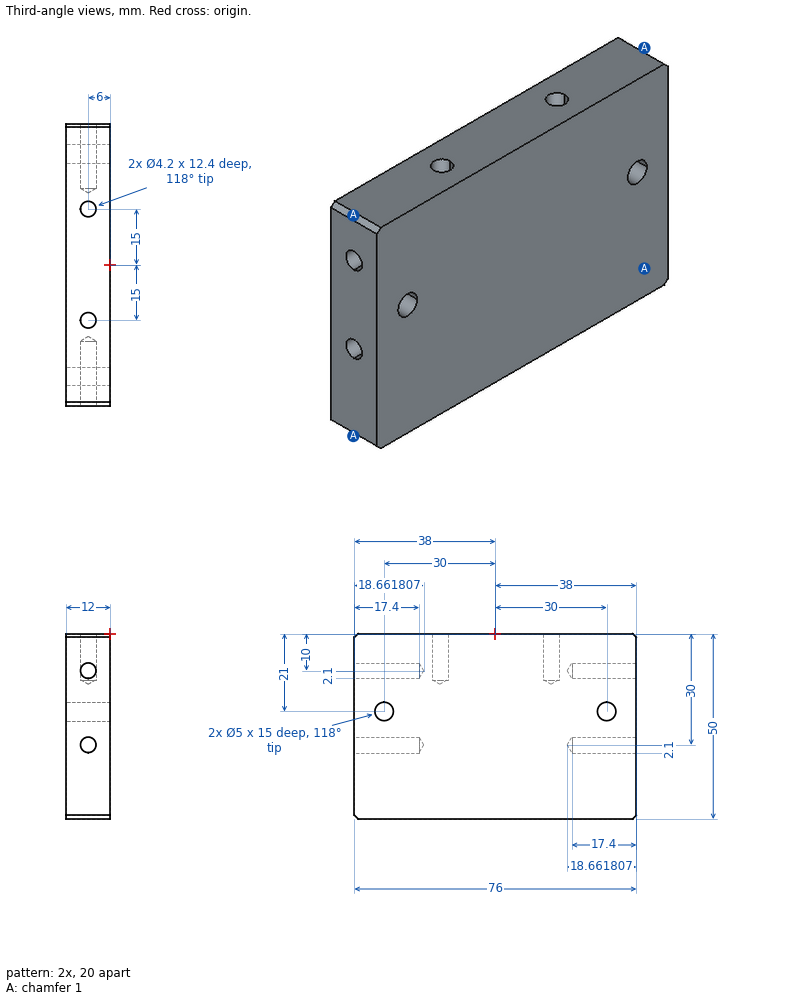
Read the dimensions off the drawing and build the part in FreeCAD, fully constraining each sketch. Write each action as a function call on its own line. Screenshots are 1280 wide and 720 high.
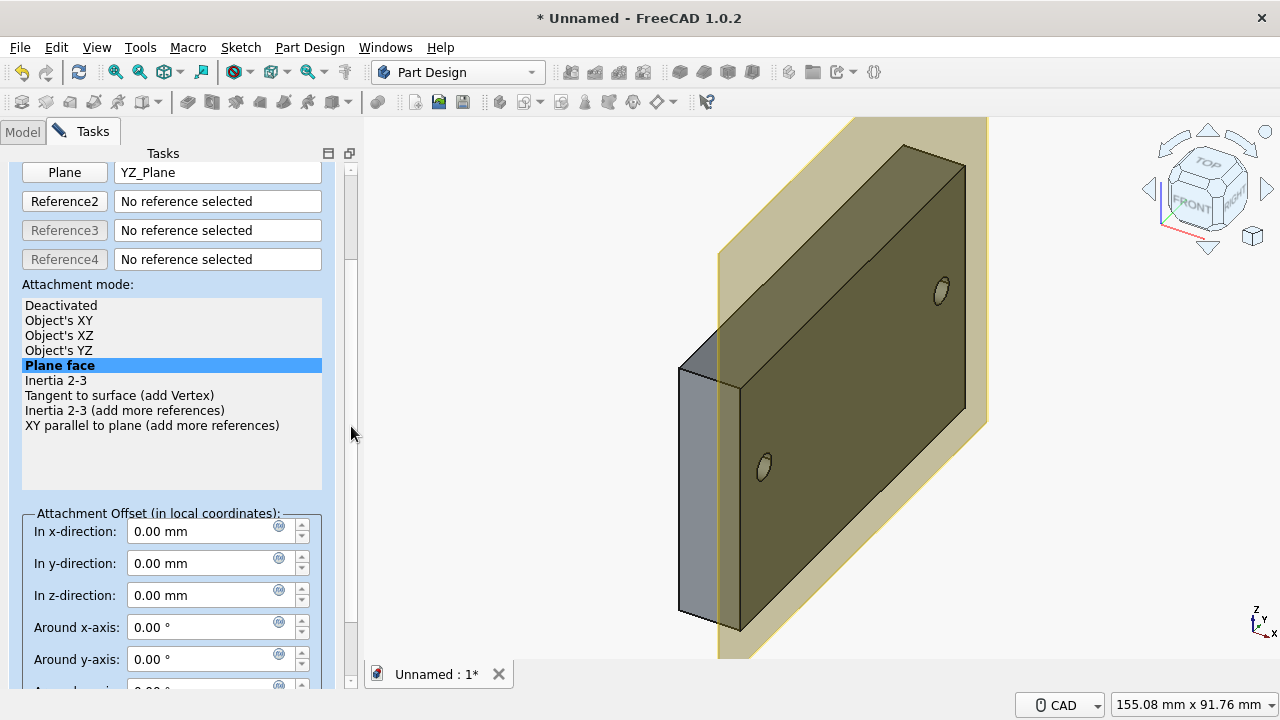
triple_click(210, 595)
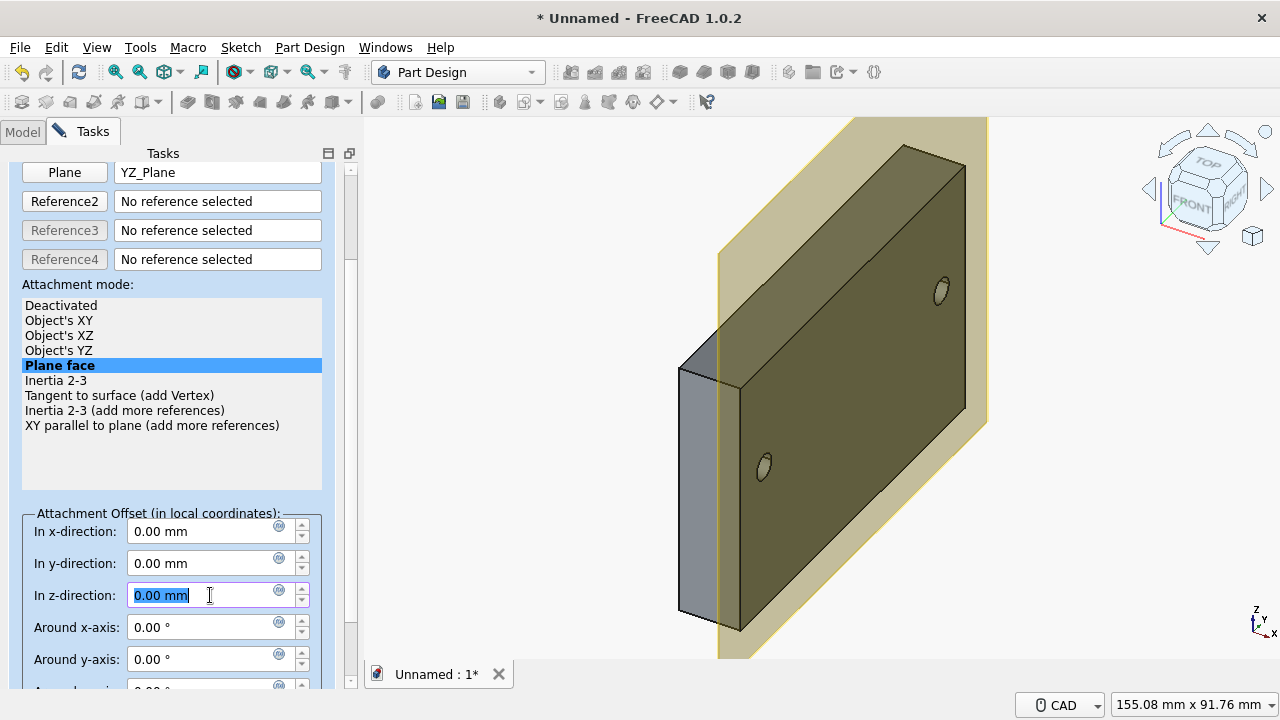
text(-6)
key(Tab)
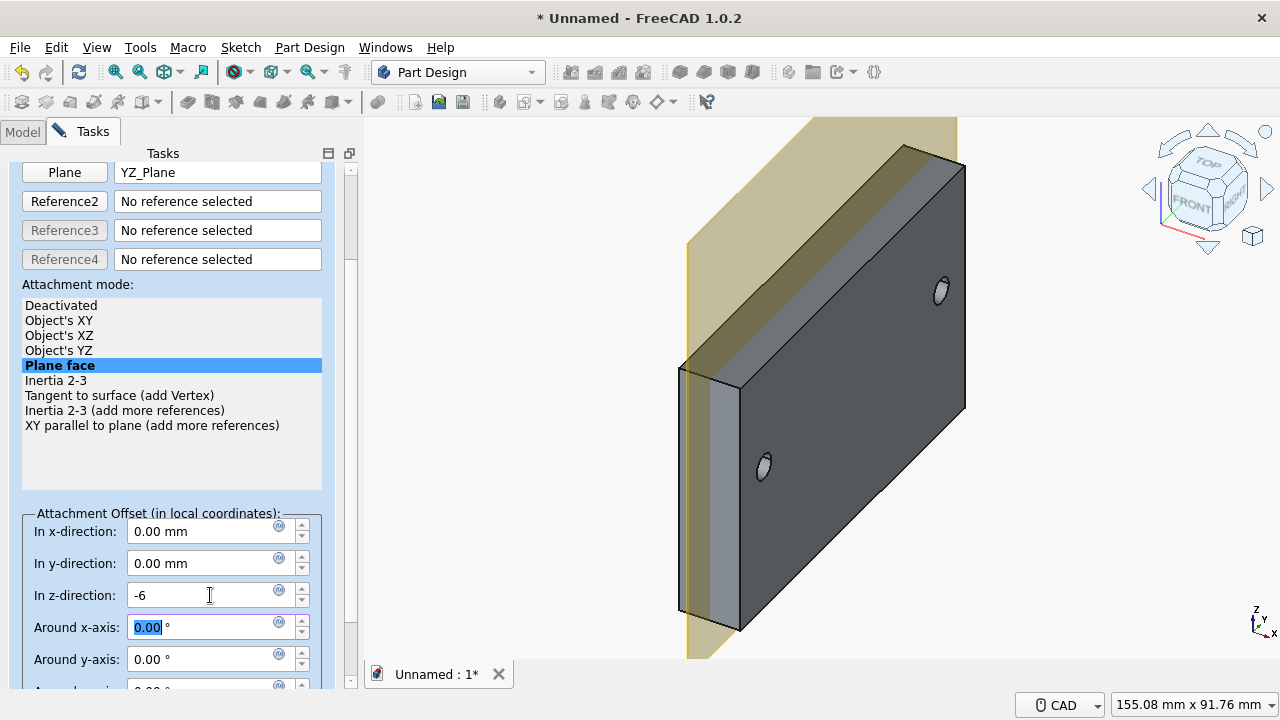
scroll(351, 426, up, 3)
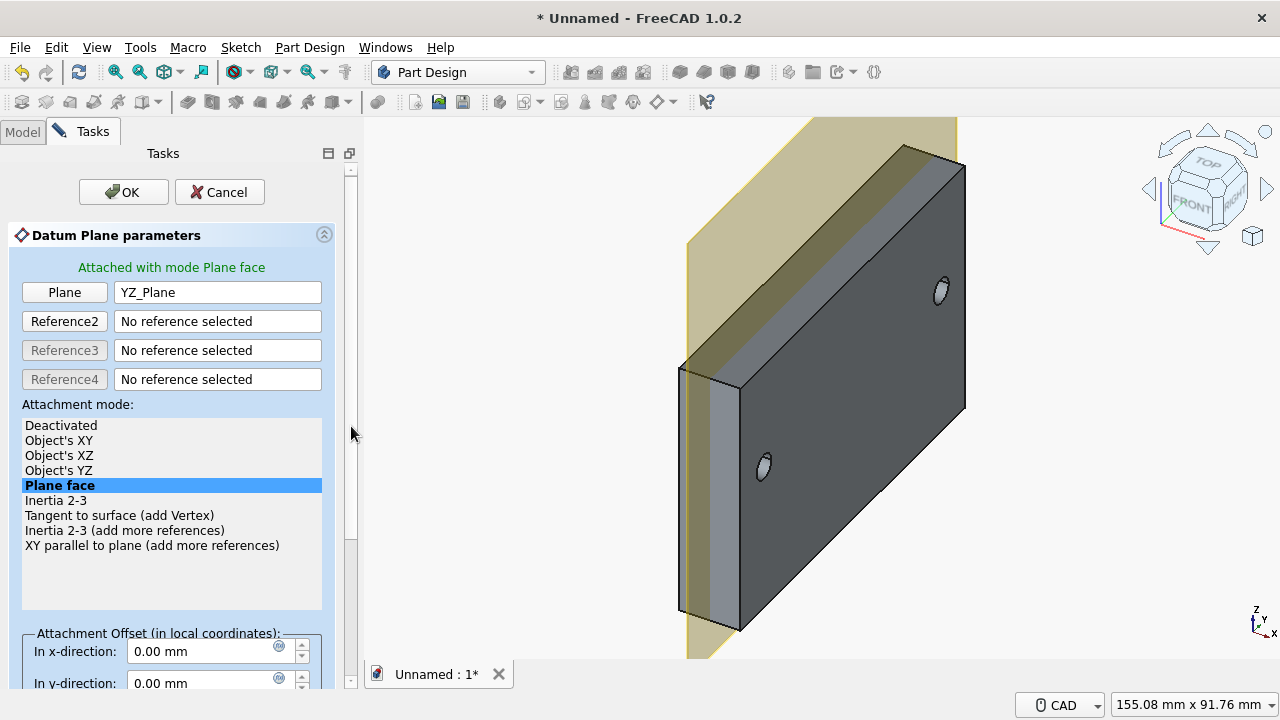
click(124, 192)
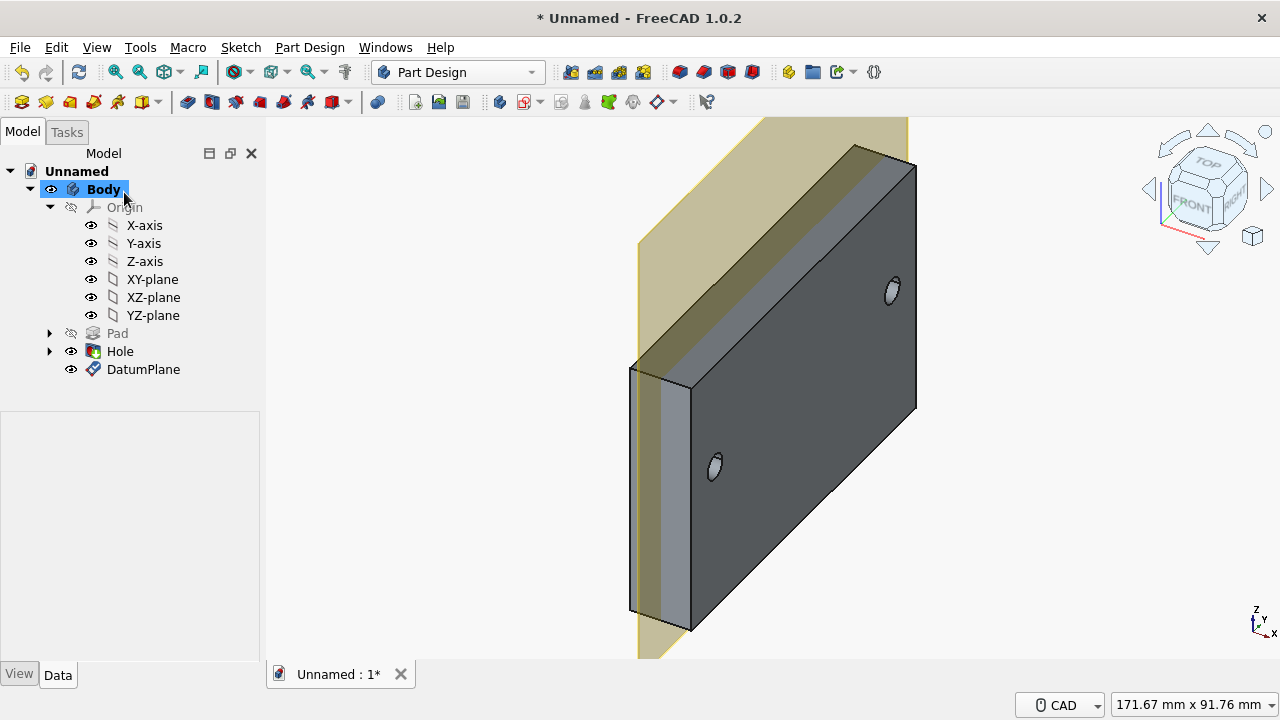
click(116, 369)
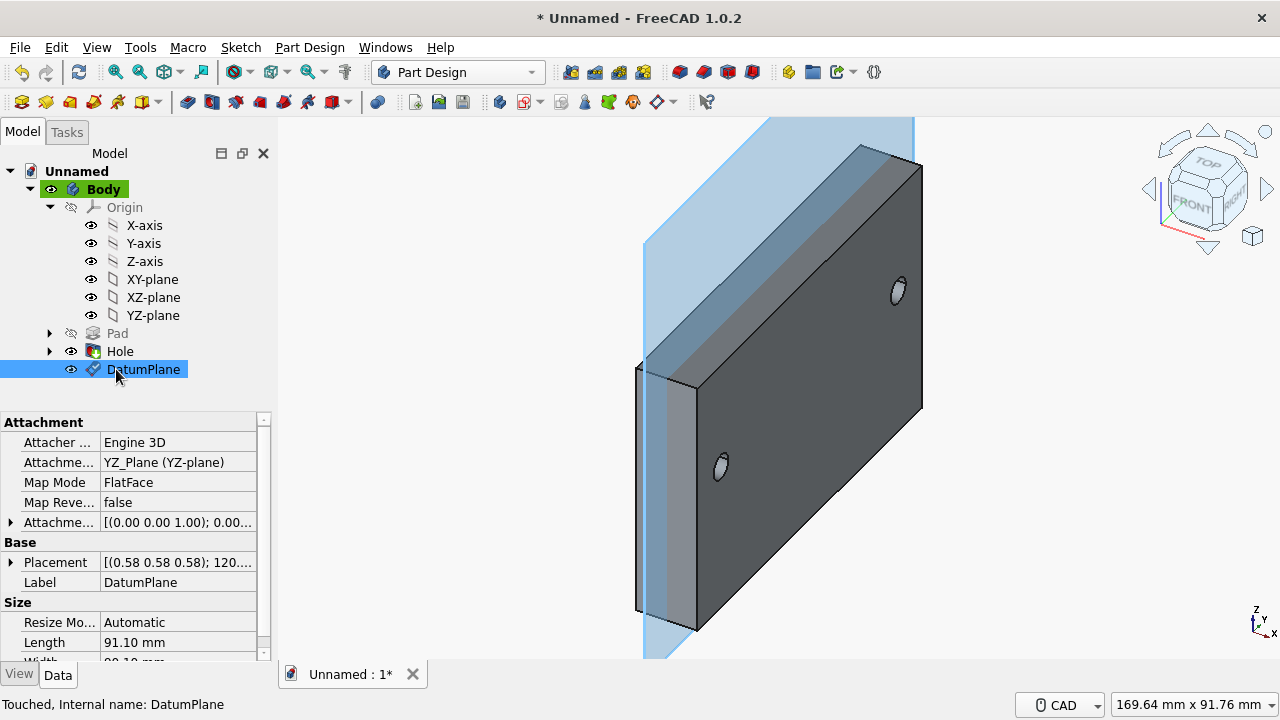
click(524, 102)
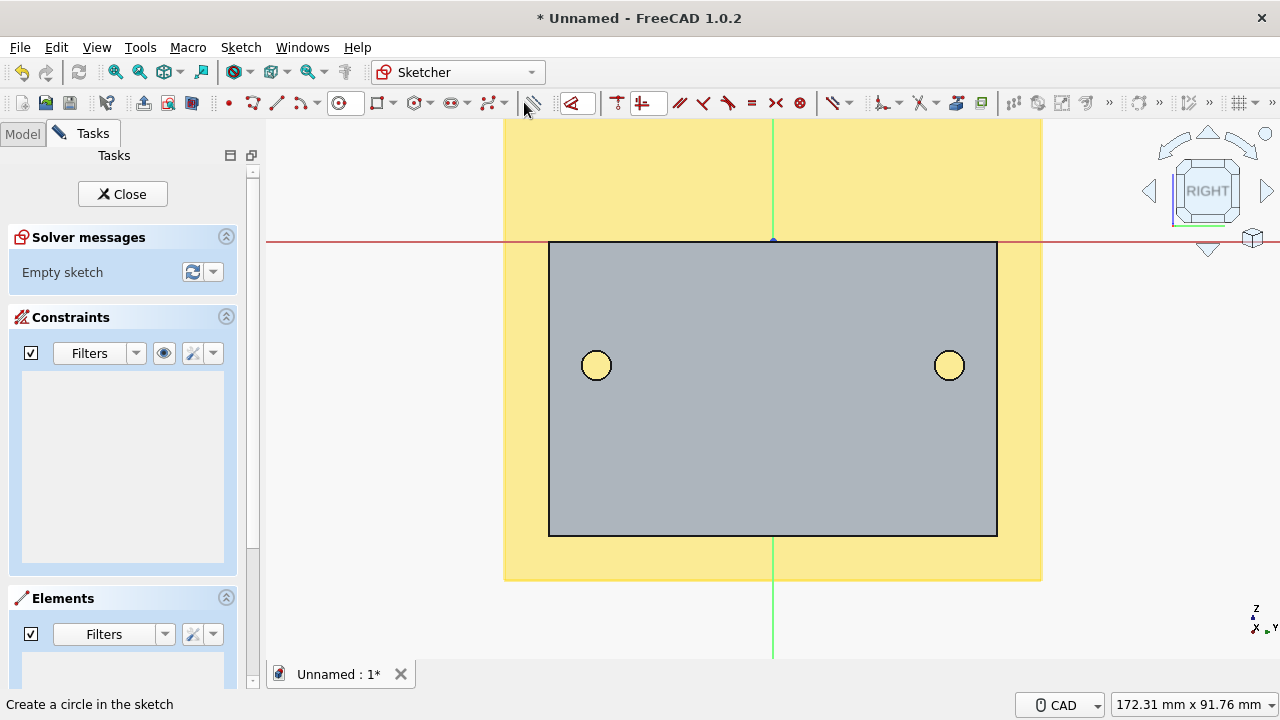
click(192, 104)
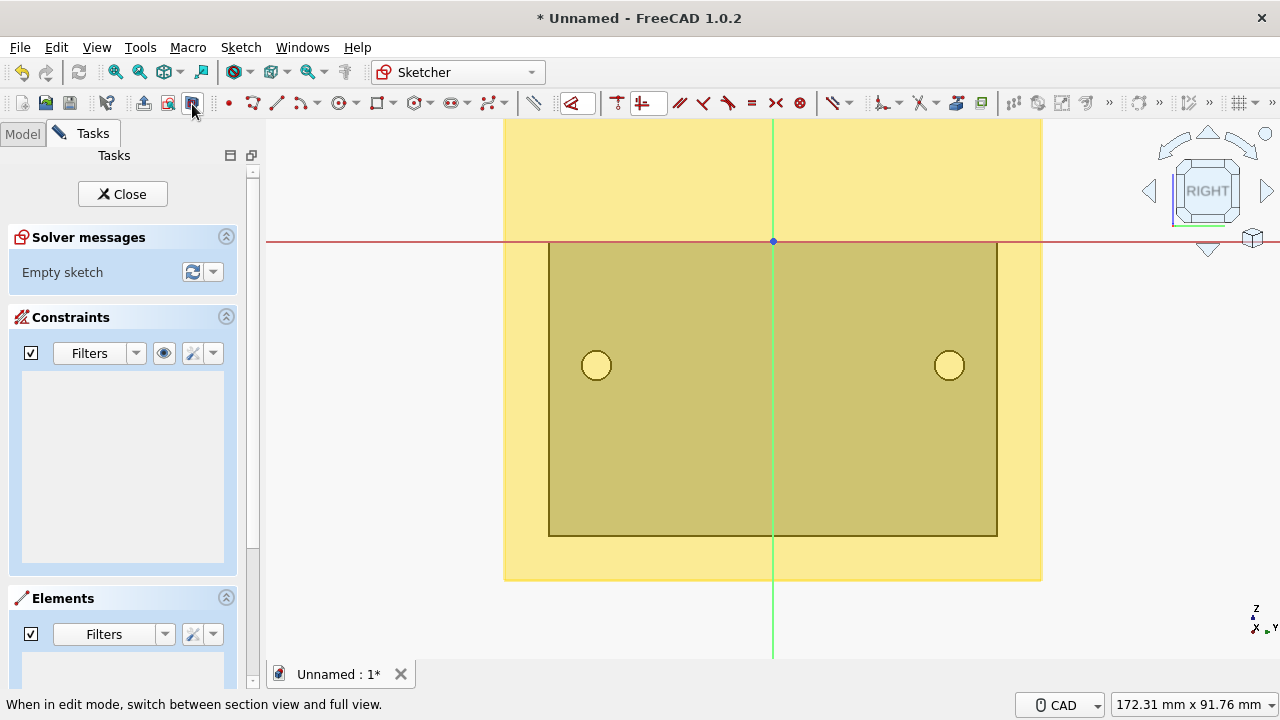
scroll(636, 213, up, 5)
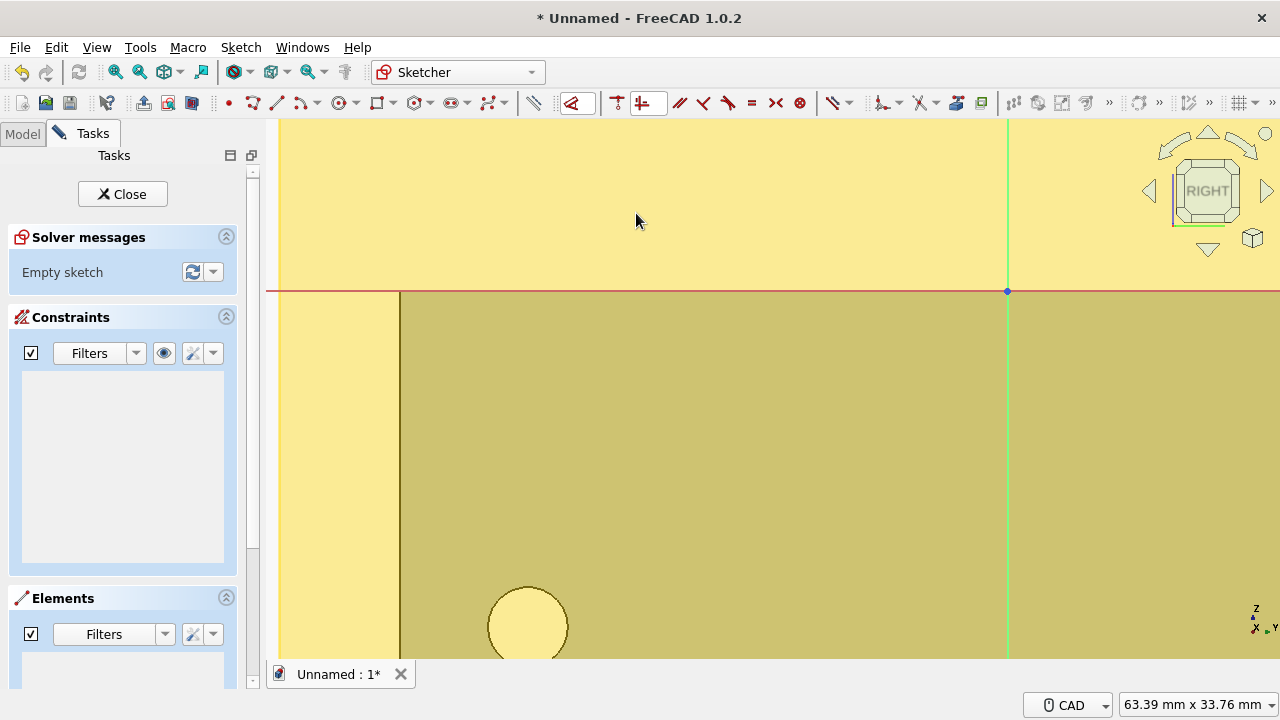
click(254, 104)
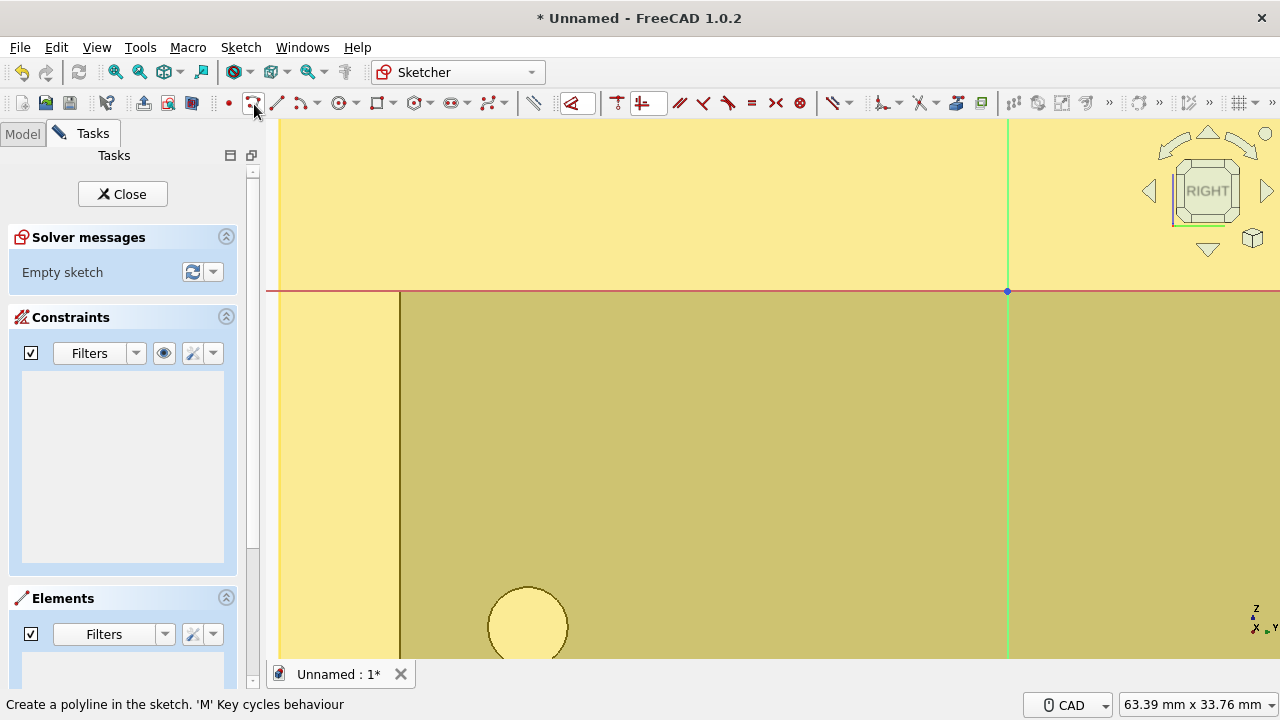
click(698, 451)
click(400, 451)
click(400, 485)
click(678, 485)
click(698, 452)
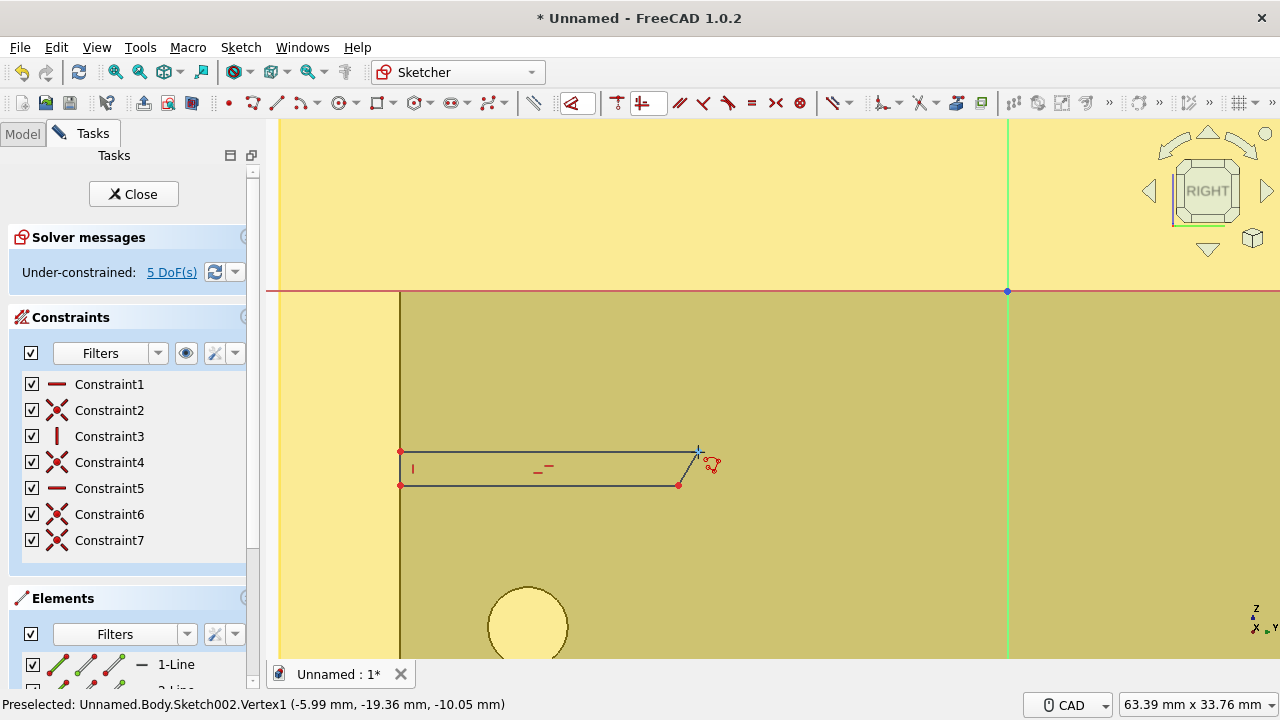
click(278, 104)